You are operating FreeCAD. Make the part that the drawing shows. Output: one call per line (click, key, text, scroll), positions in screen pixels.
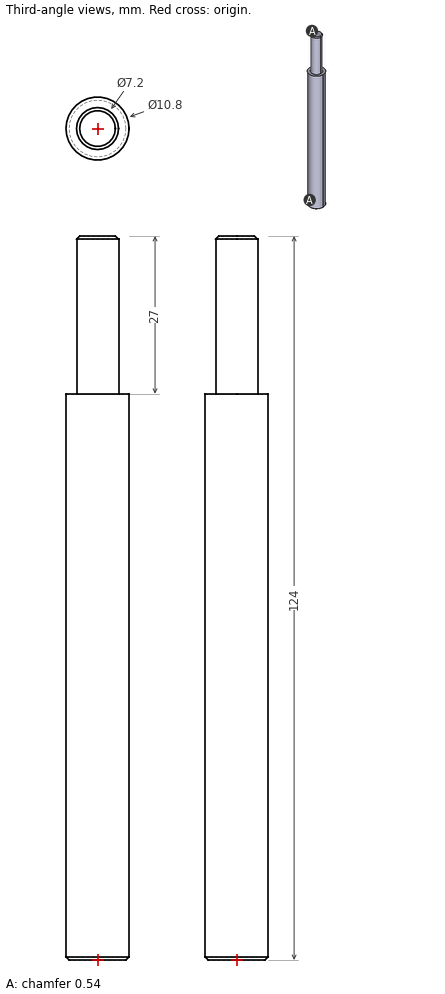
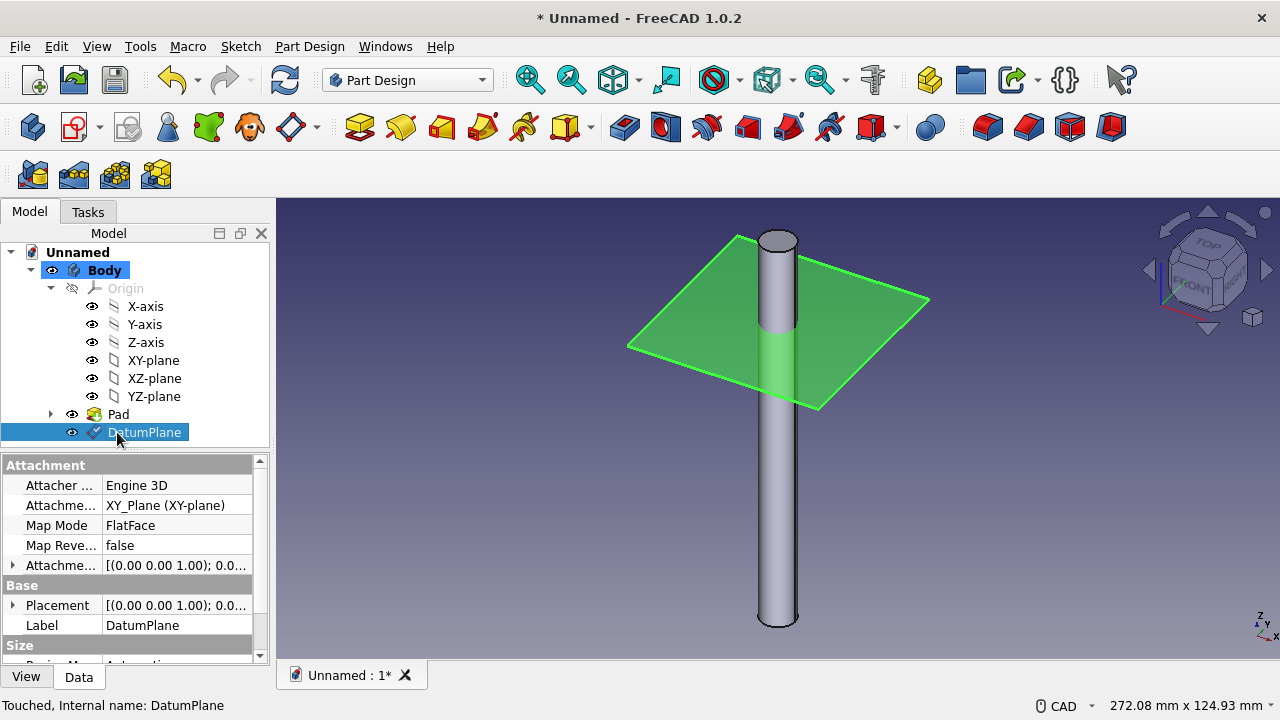
click(74, 128)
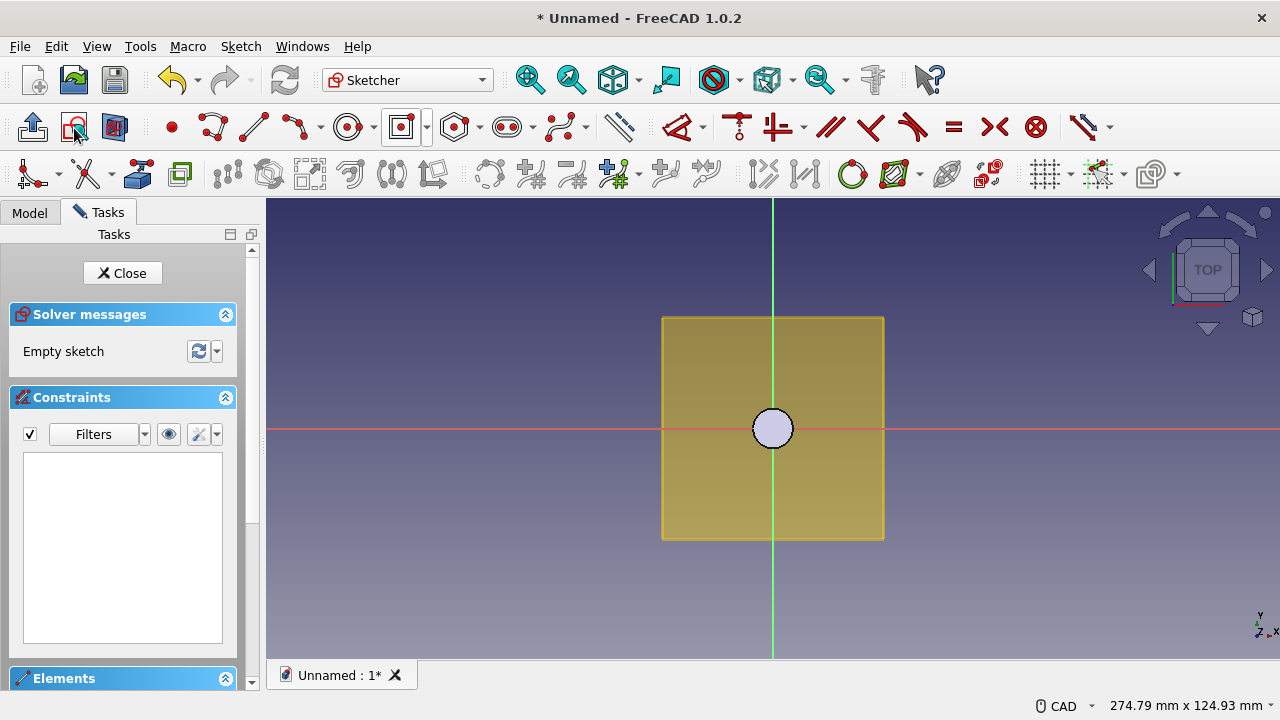
click(115, 128)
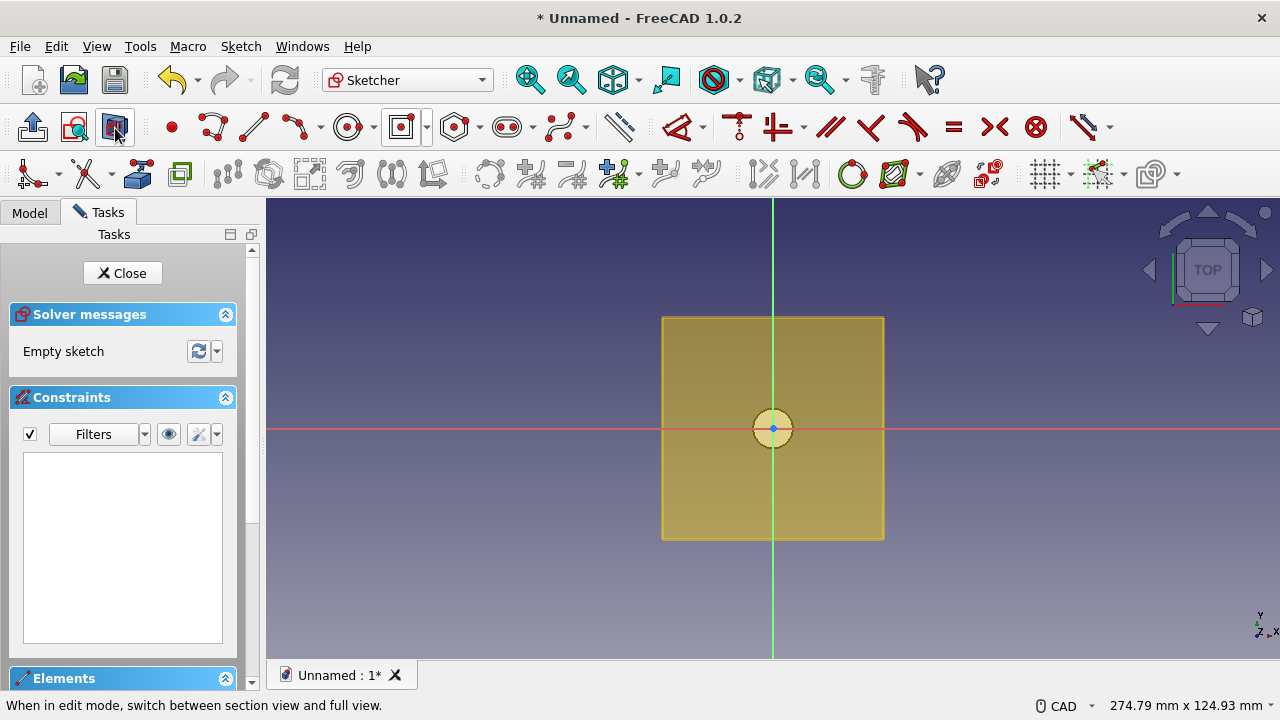
scroll(784, 428, up, 10)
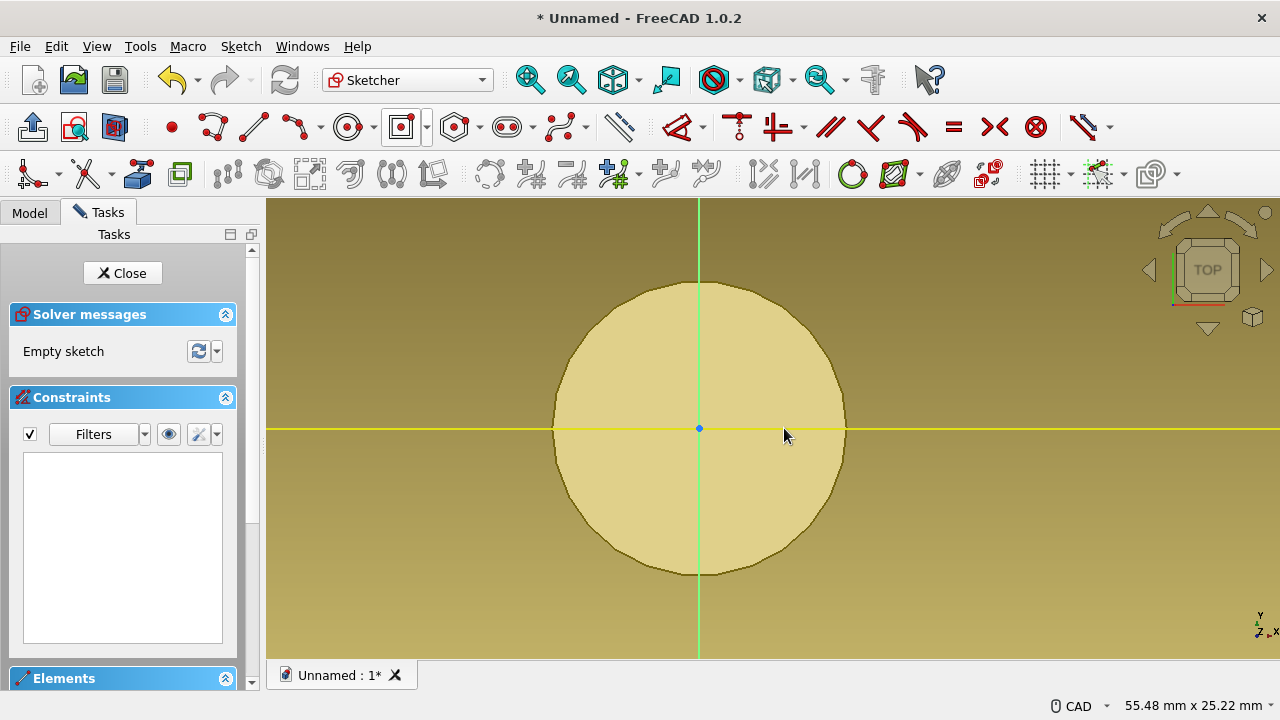
click(348, 128)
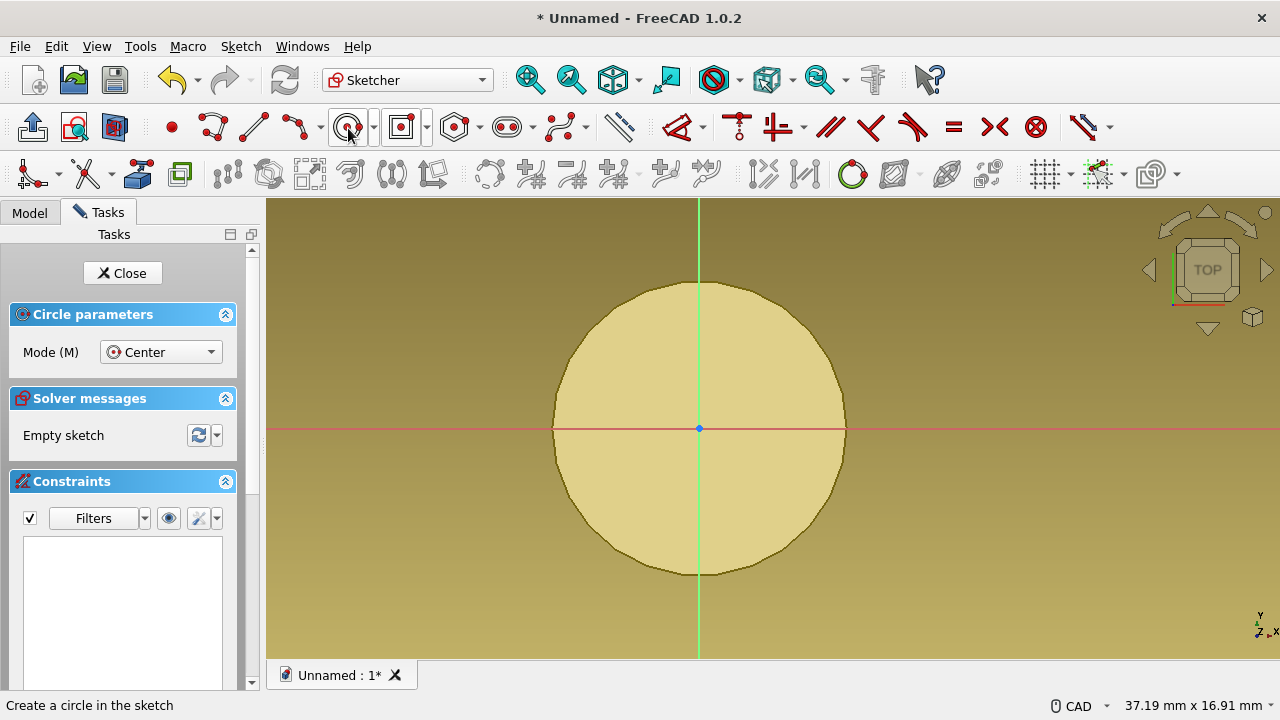
click(699, 428)
click(804, 324)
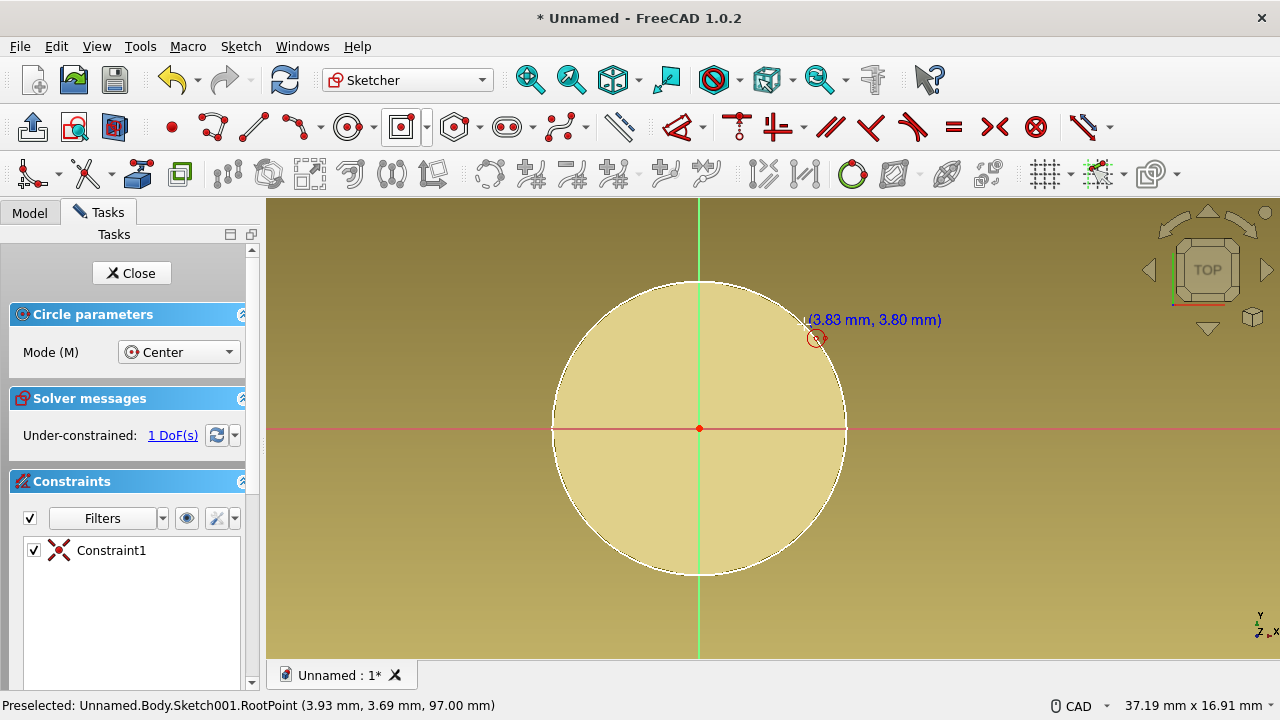
click(699, 428)
click(769, 359)
key(Escape)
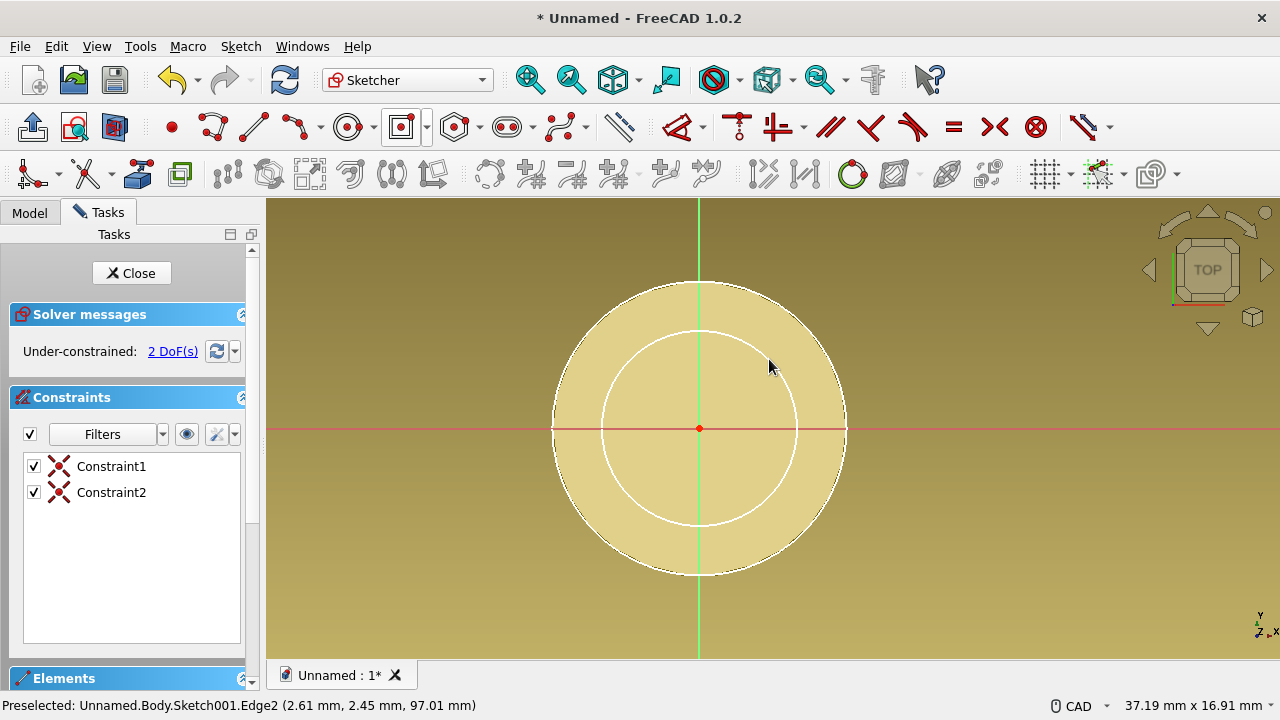
key(d)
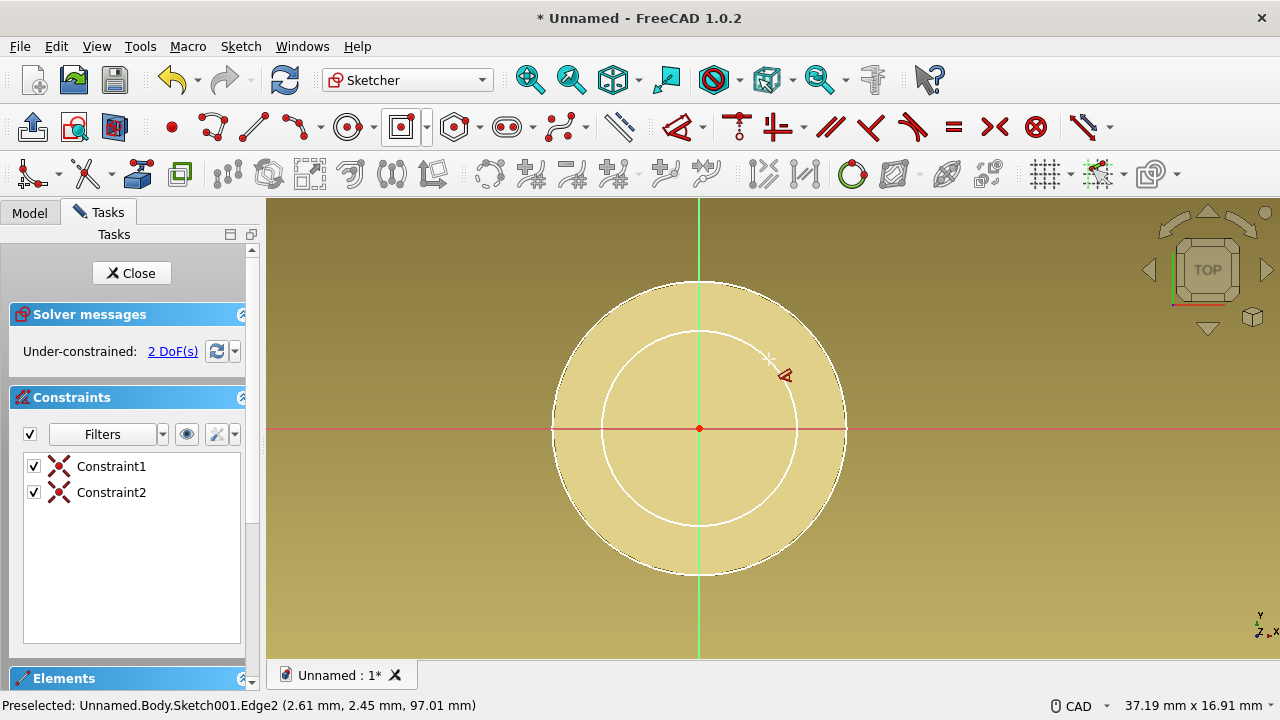
click(803, 324)
click(826, 301)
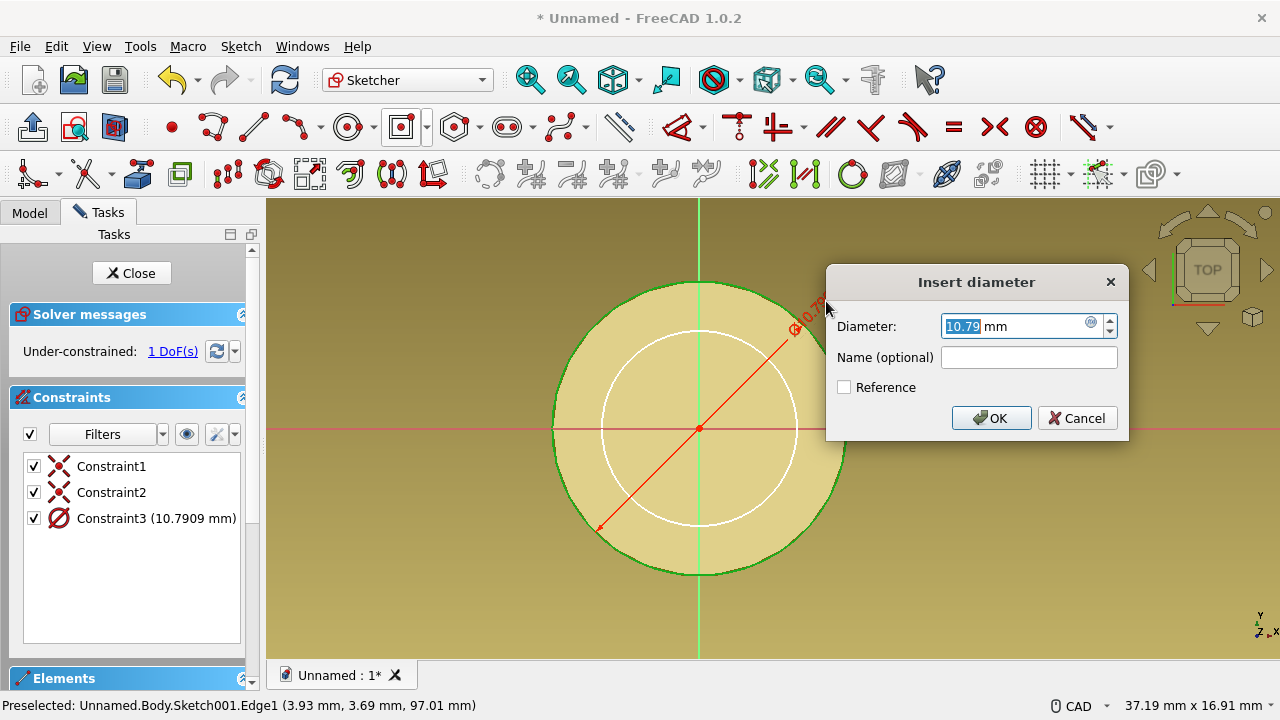
text(10.8)
key(Return)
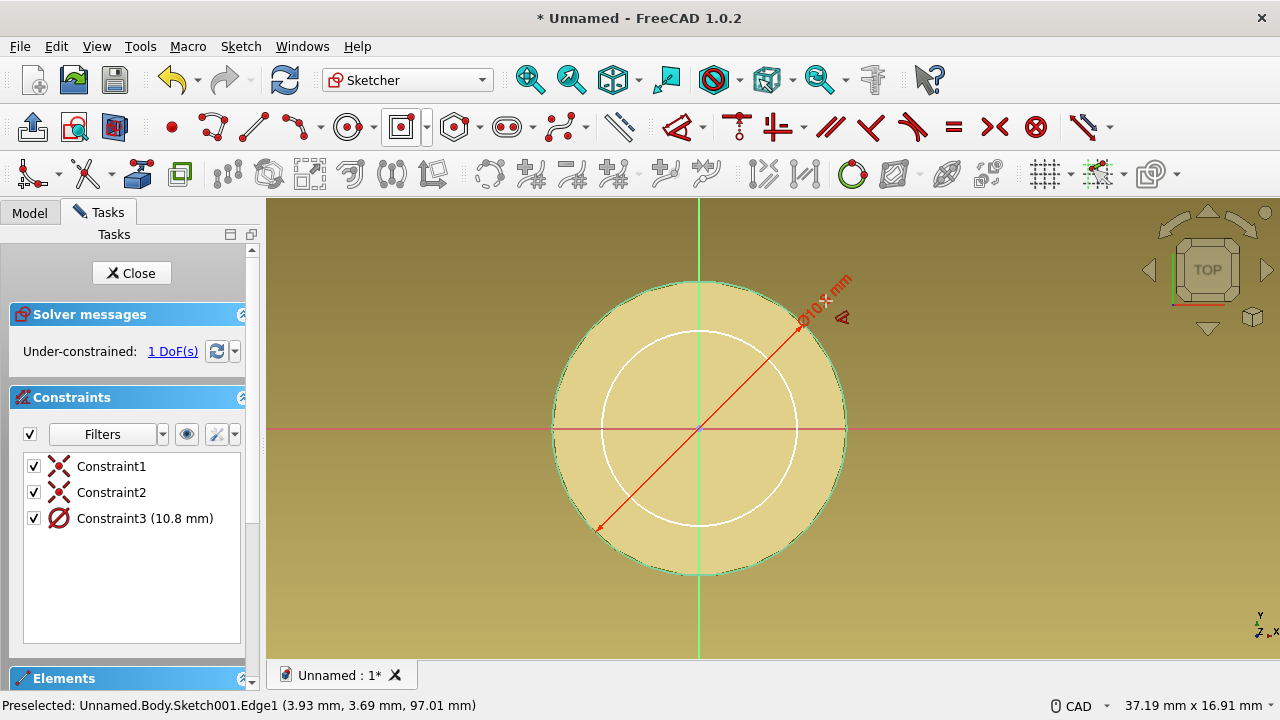
click(768, 359)
click(790, 336)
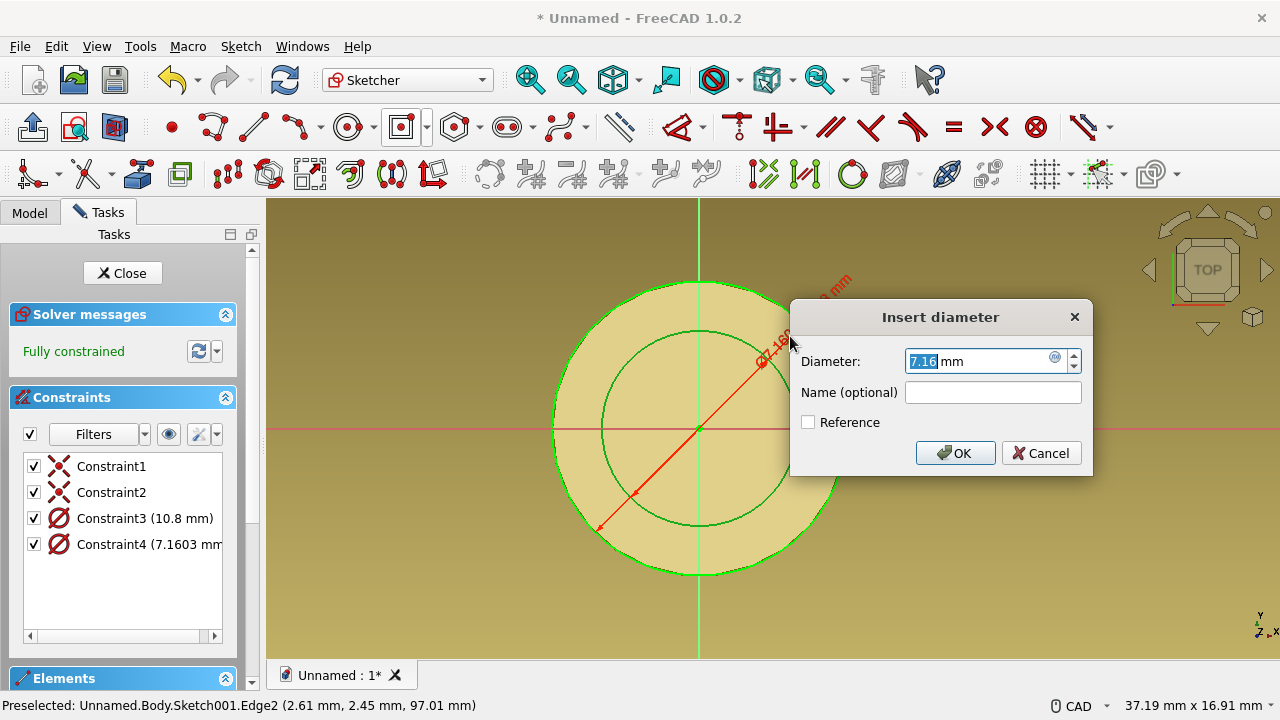
text(7.2)
key(Return)
key(Escape)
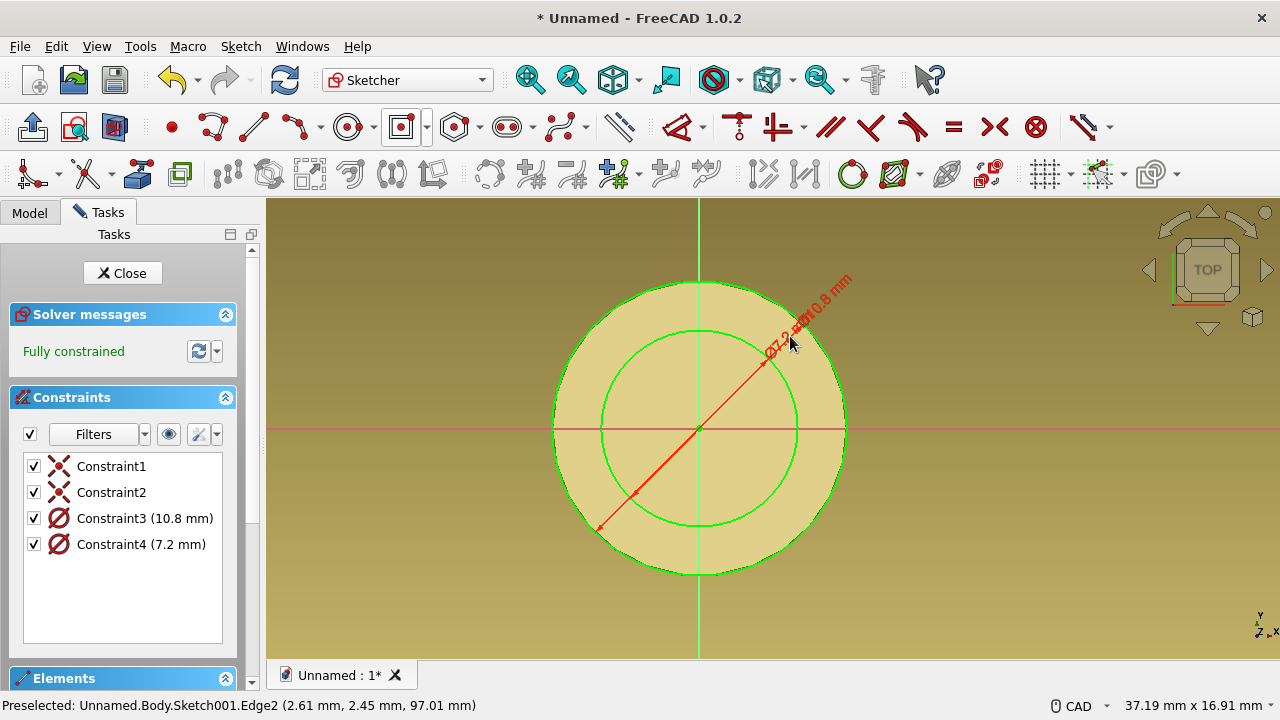
click(123, 273)